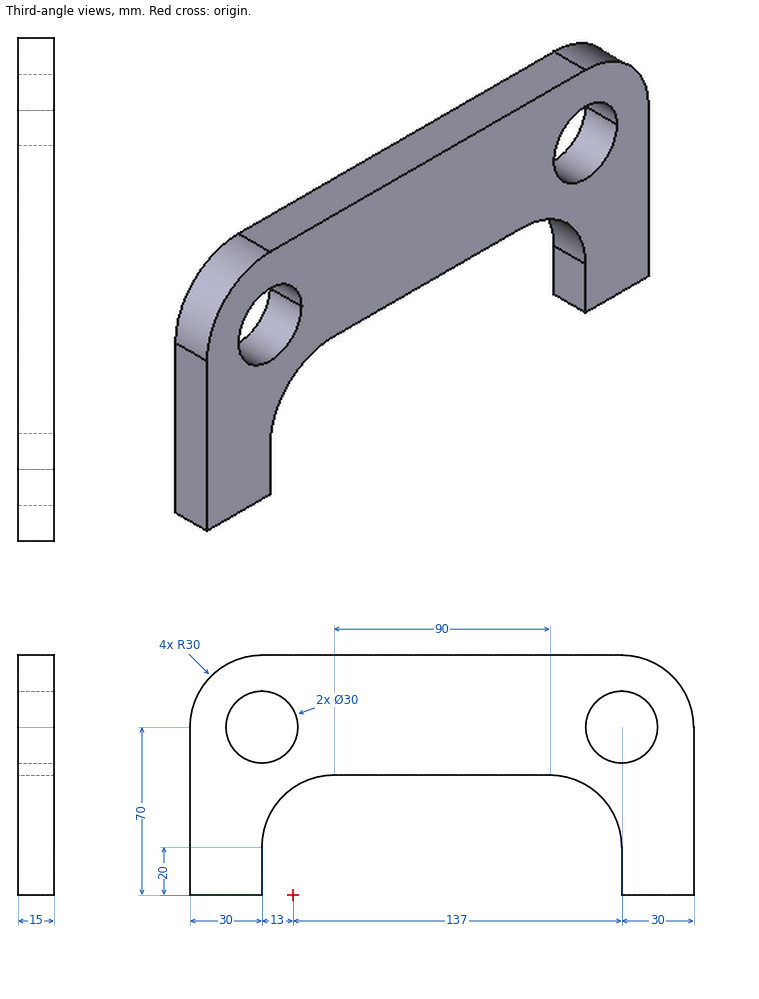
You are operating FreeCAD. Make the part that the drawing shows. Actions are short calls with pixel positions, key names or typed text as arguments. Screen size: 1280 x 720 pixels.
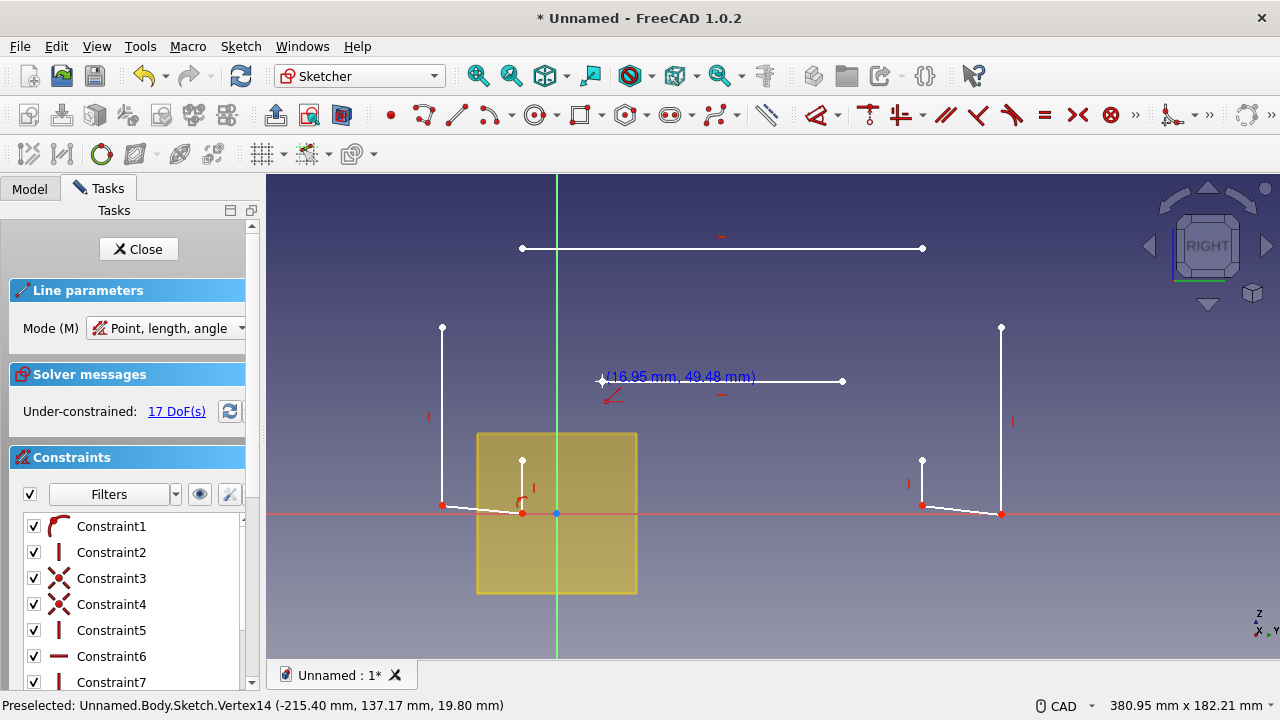
key(g)
key(3)
key(a)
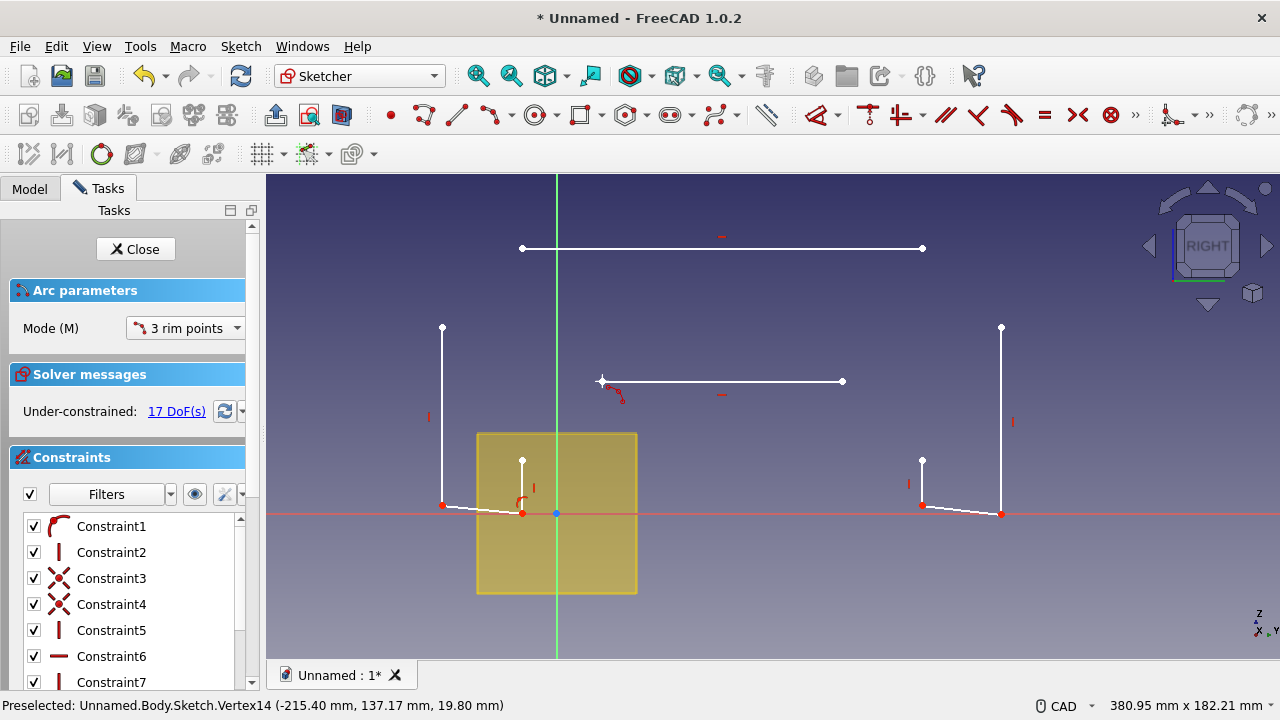
click(442, 328)
click(522, 249)
click(466, 271)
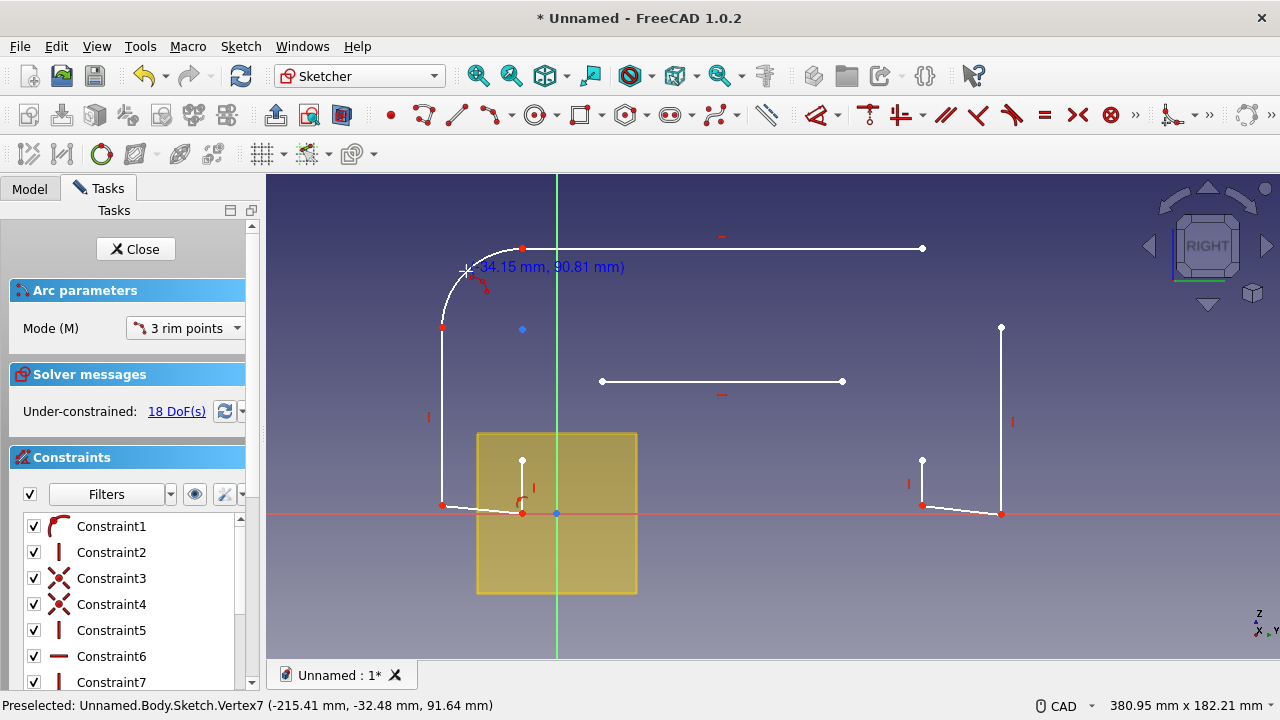
click(922, 249)
click(1001, 328)
click(978, 271)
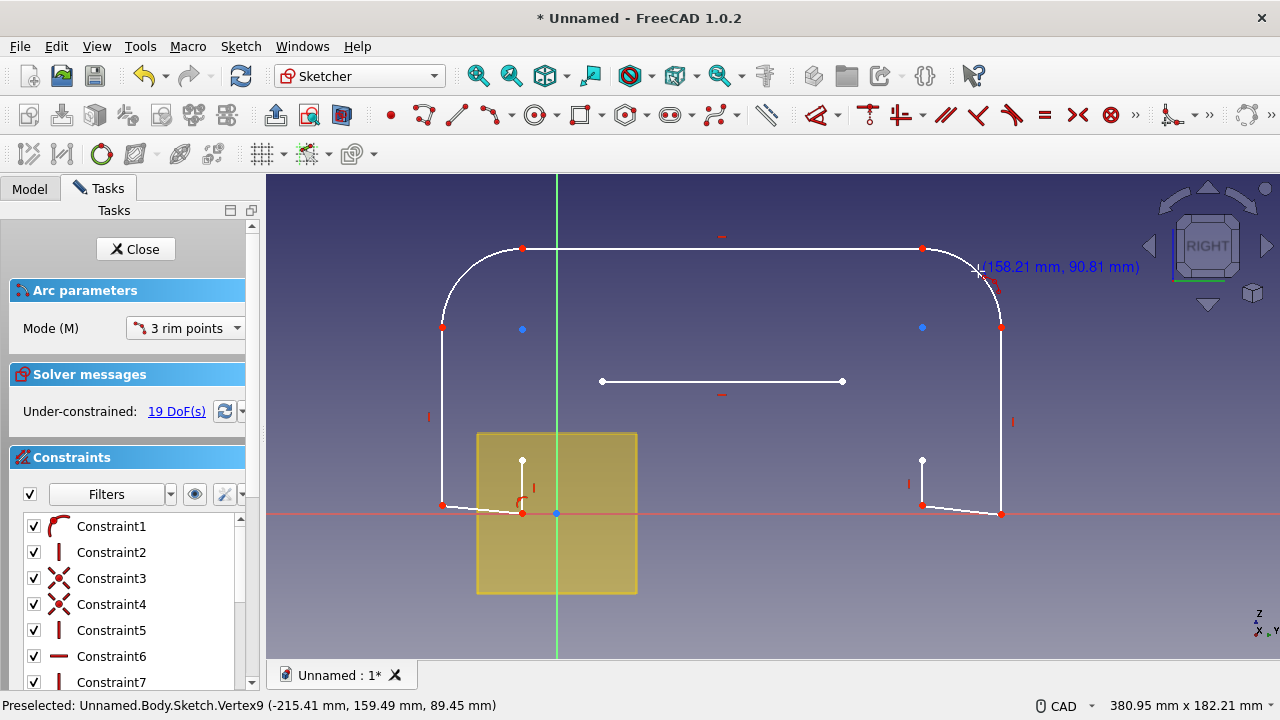
click(922, 461)
click(842, 382)
click(898, 404)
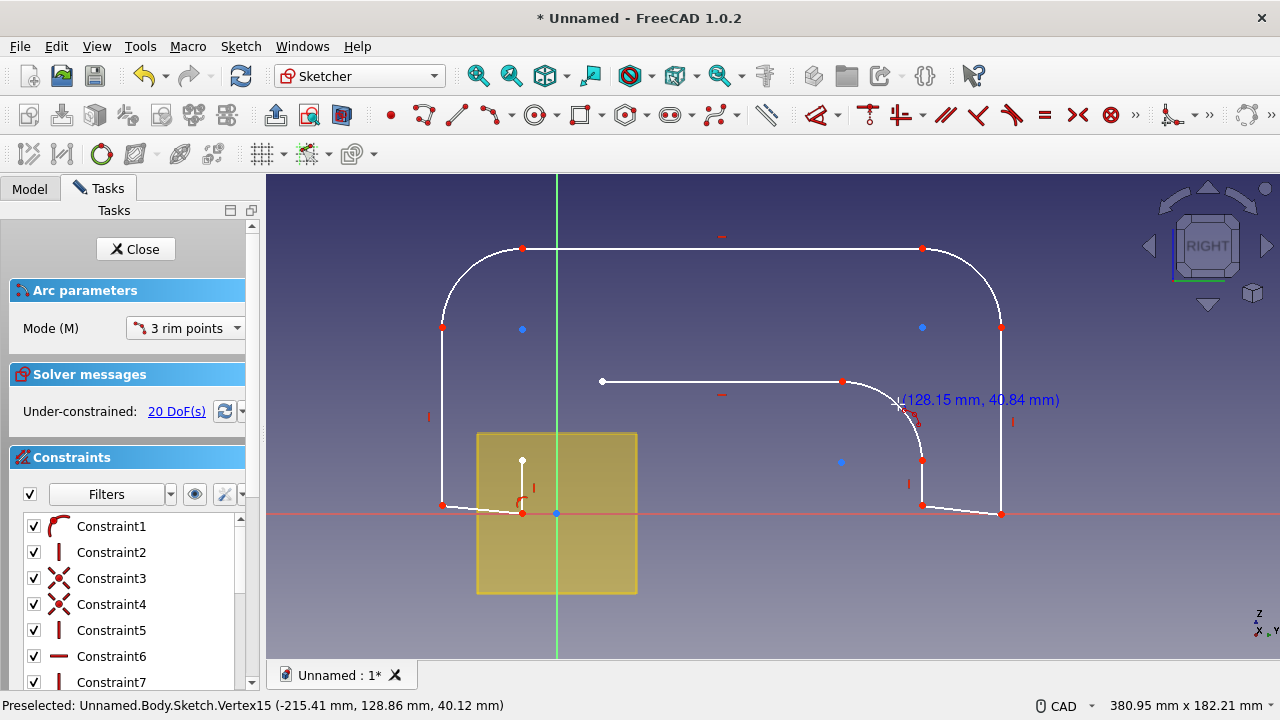
click(602, 382)
click(522, 461)
click(538, 414)
key(Escape)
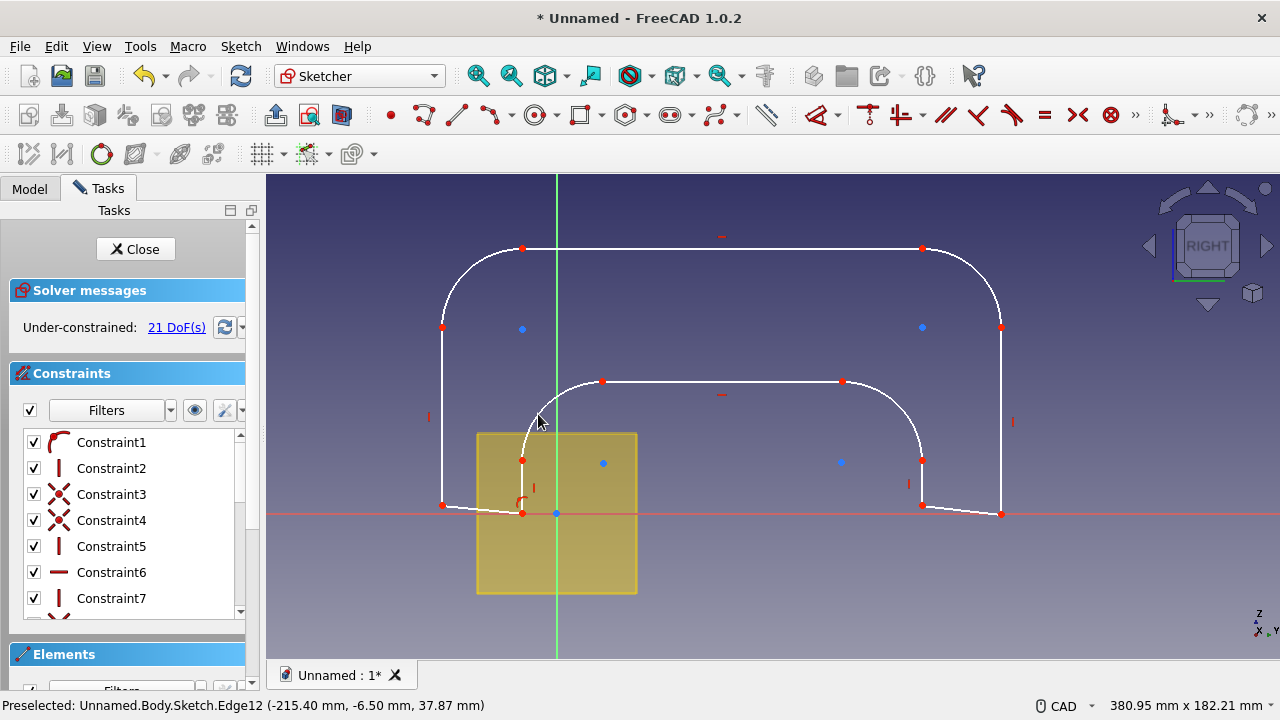
click(522, 477)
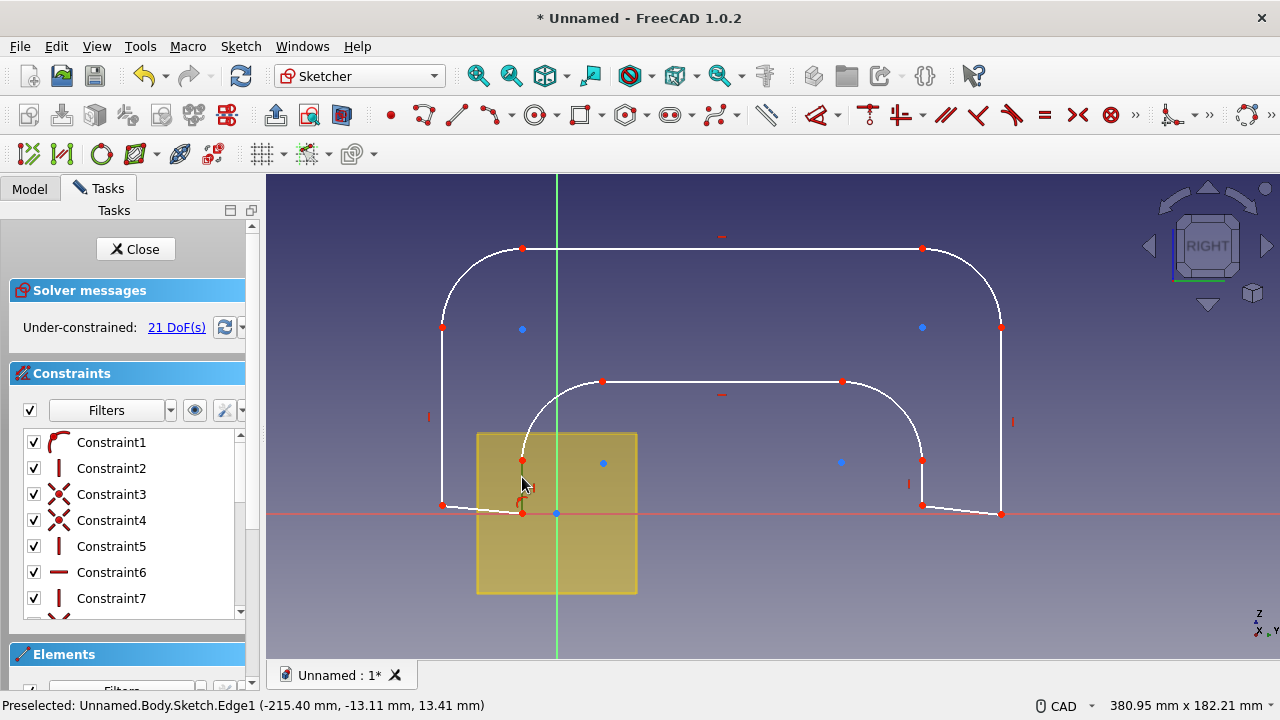
scroll(566, 391, up, 2)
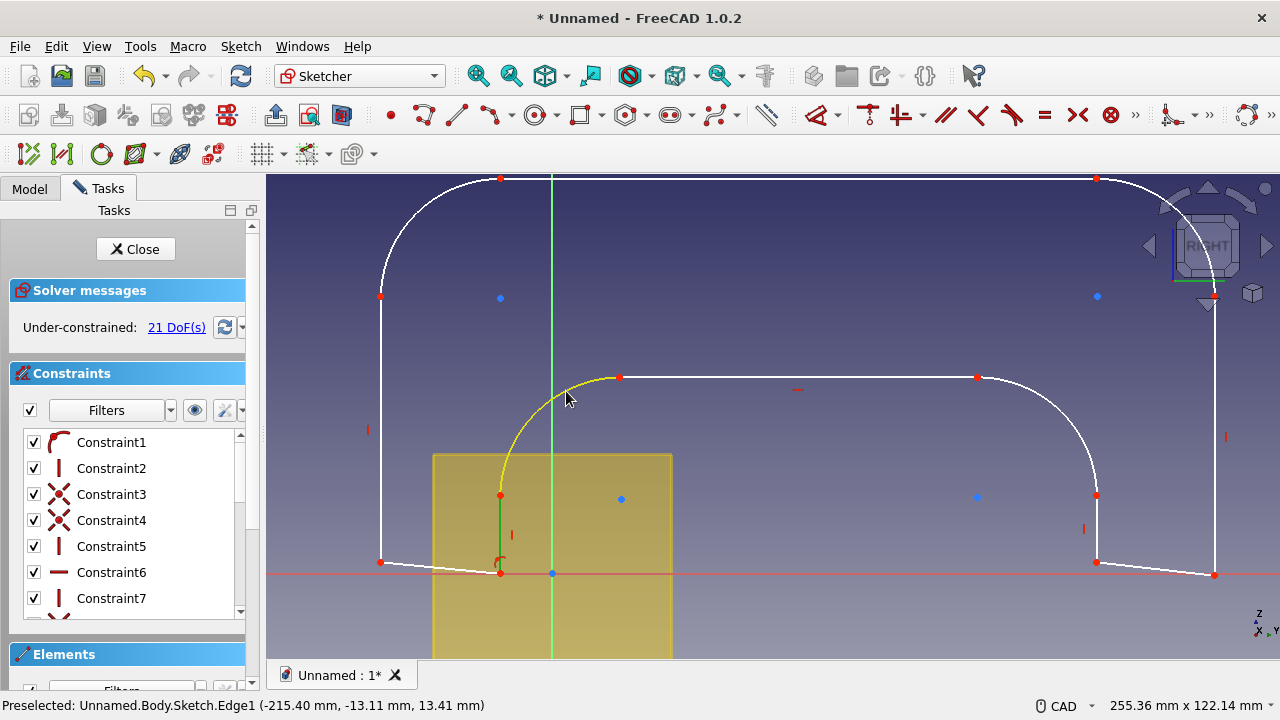
click(566, 391)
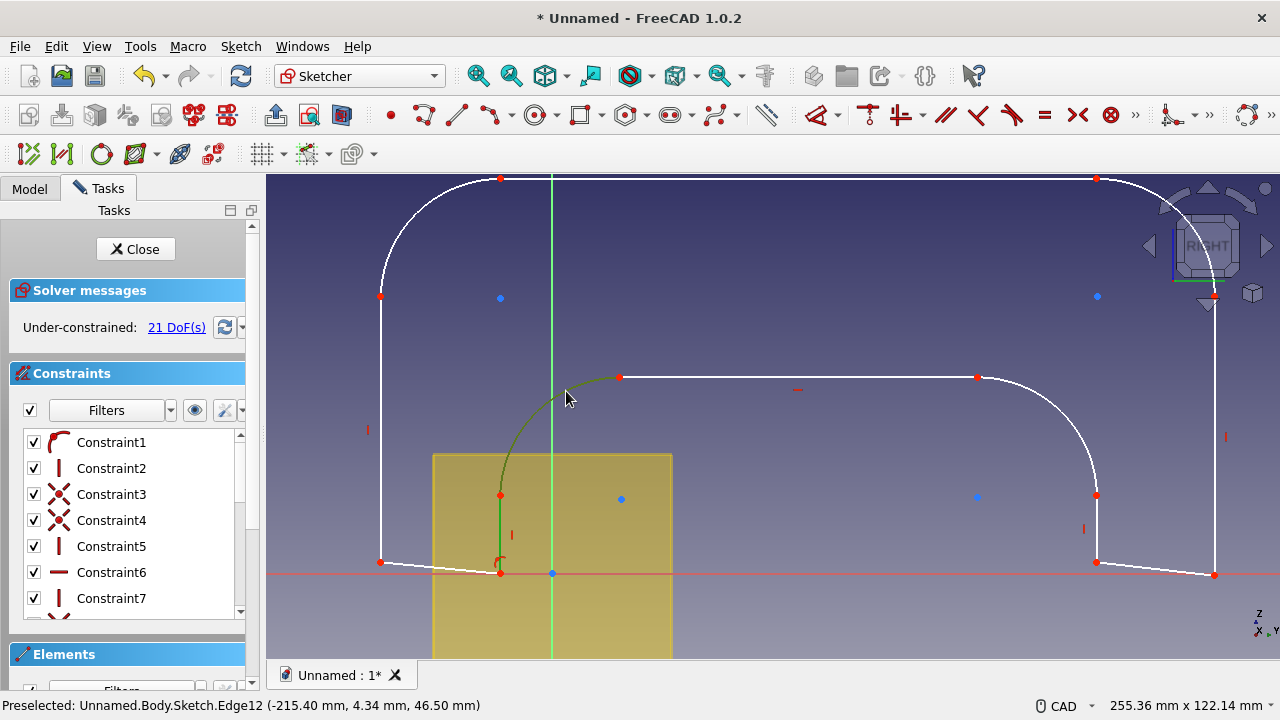
key(t)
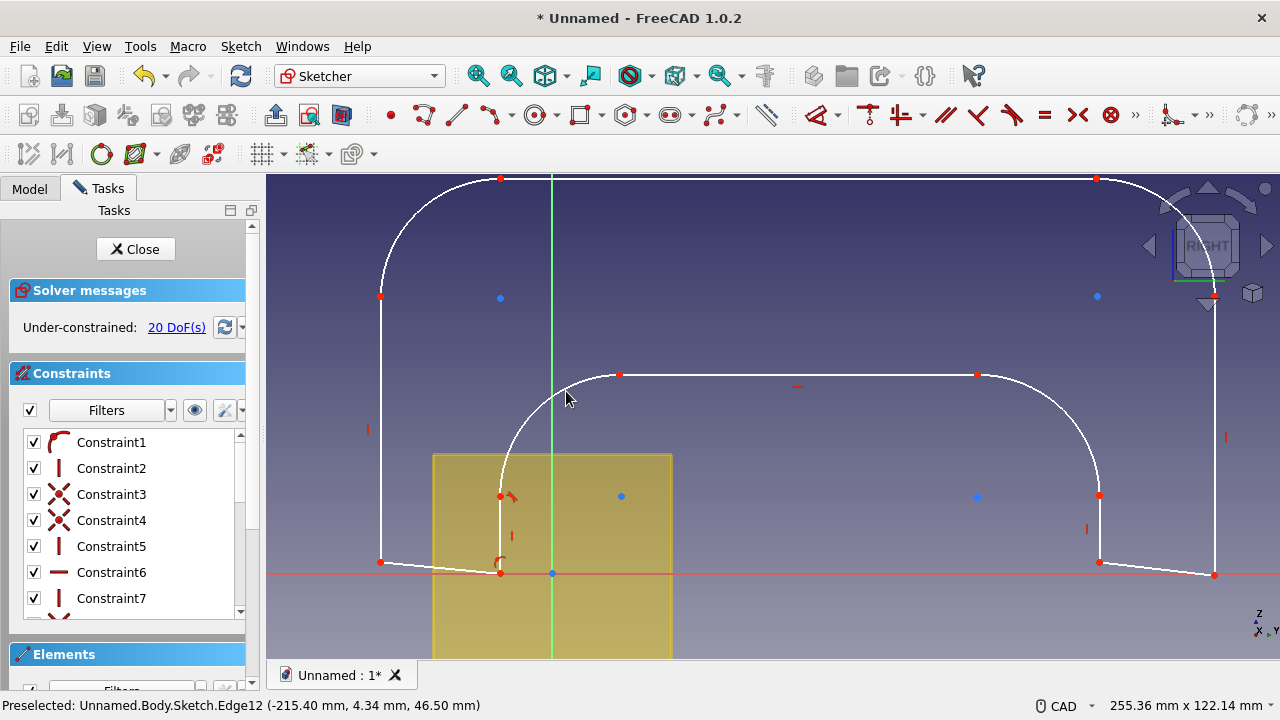
click(381, 483)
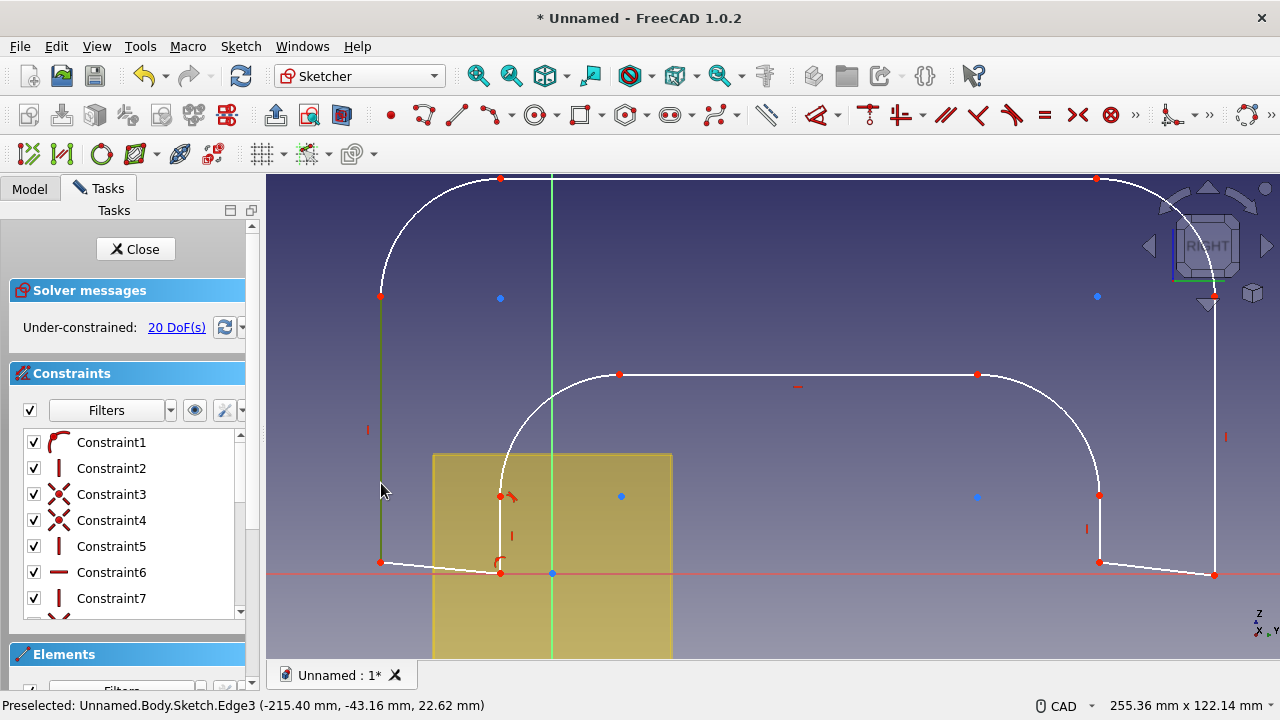
click(394, 243)